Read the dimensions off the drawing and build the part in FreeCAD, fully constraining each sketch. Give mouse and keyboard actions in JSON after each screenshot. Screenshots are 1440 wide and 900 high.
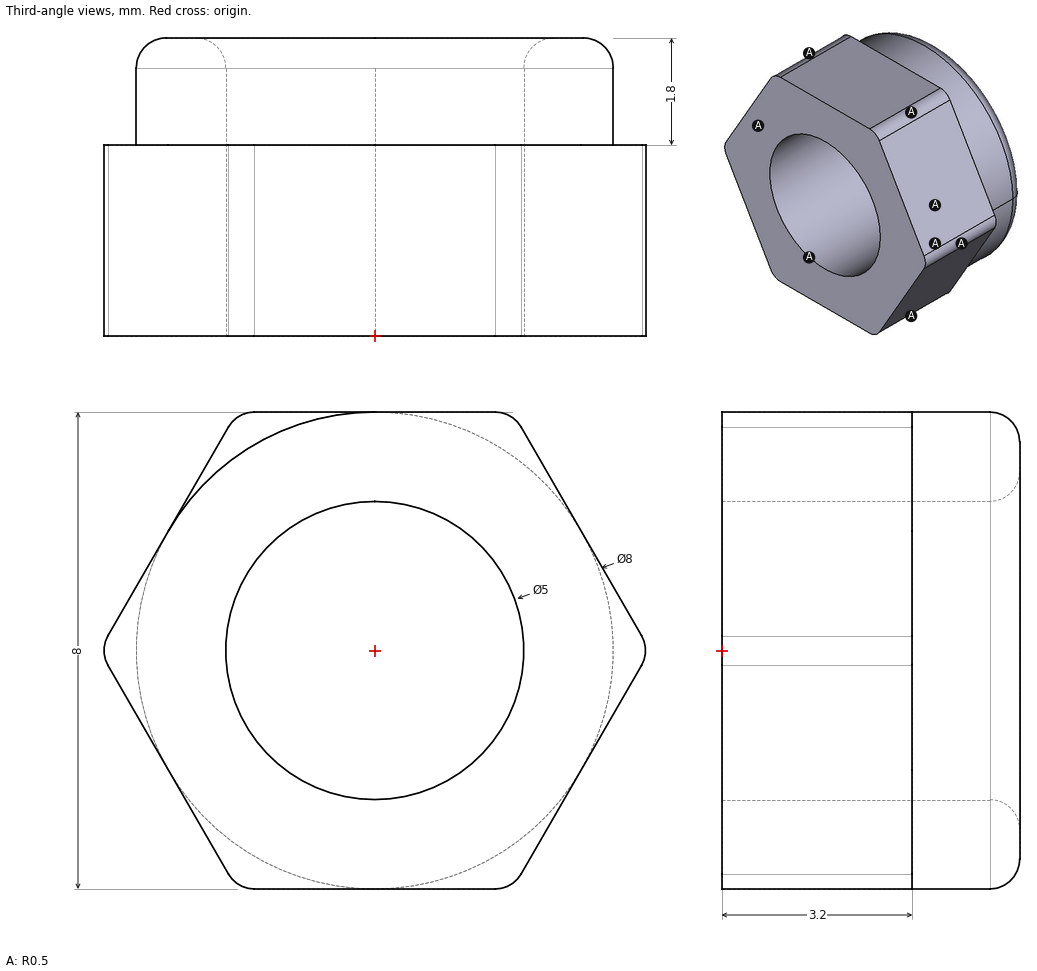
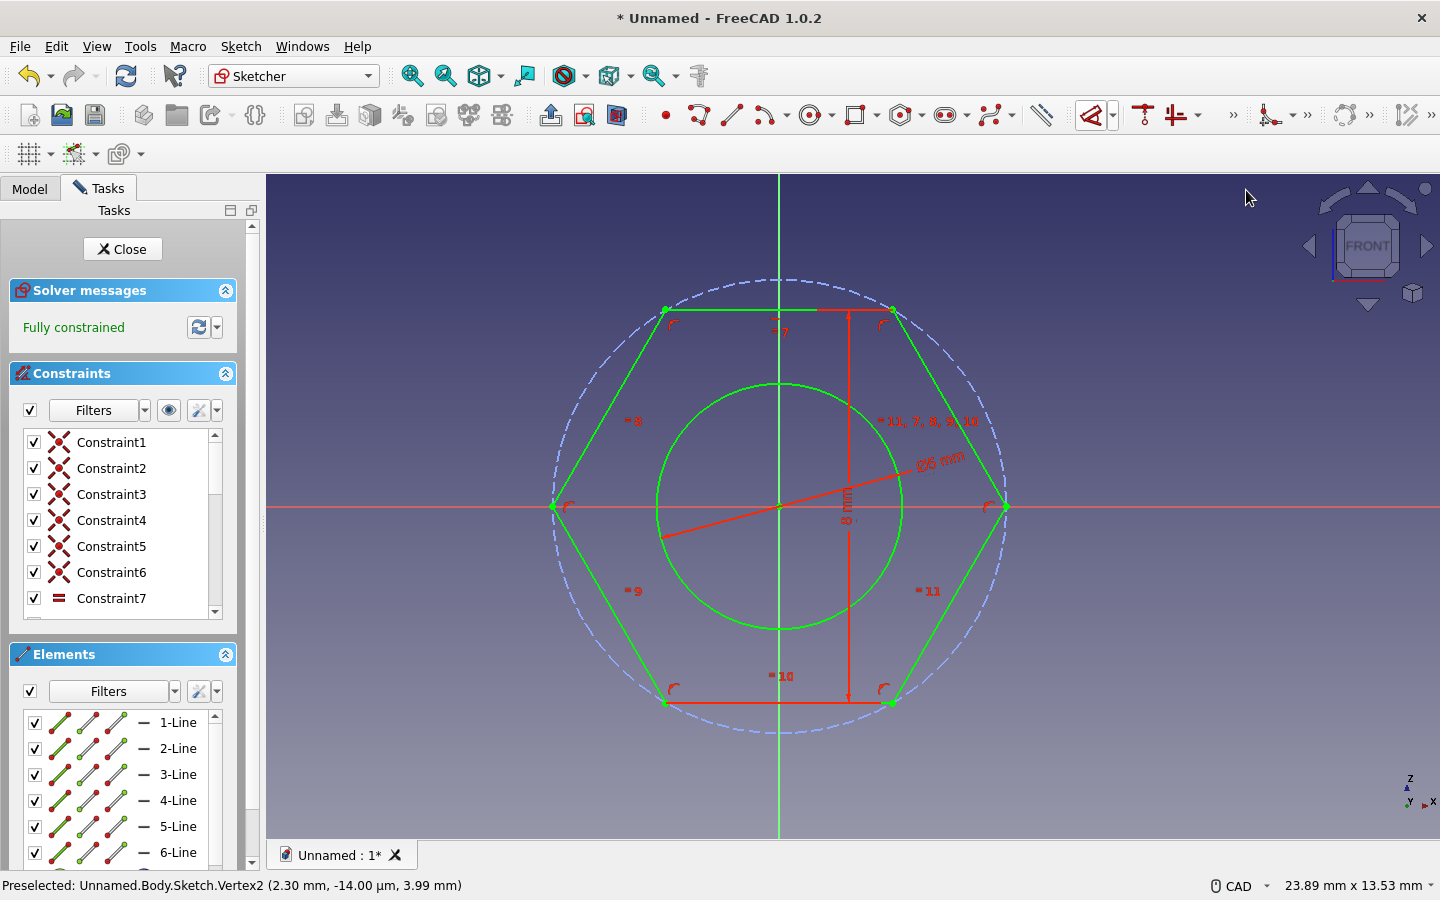
{"action": "left_click", "coordinate": [123, 249]}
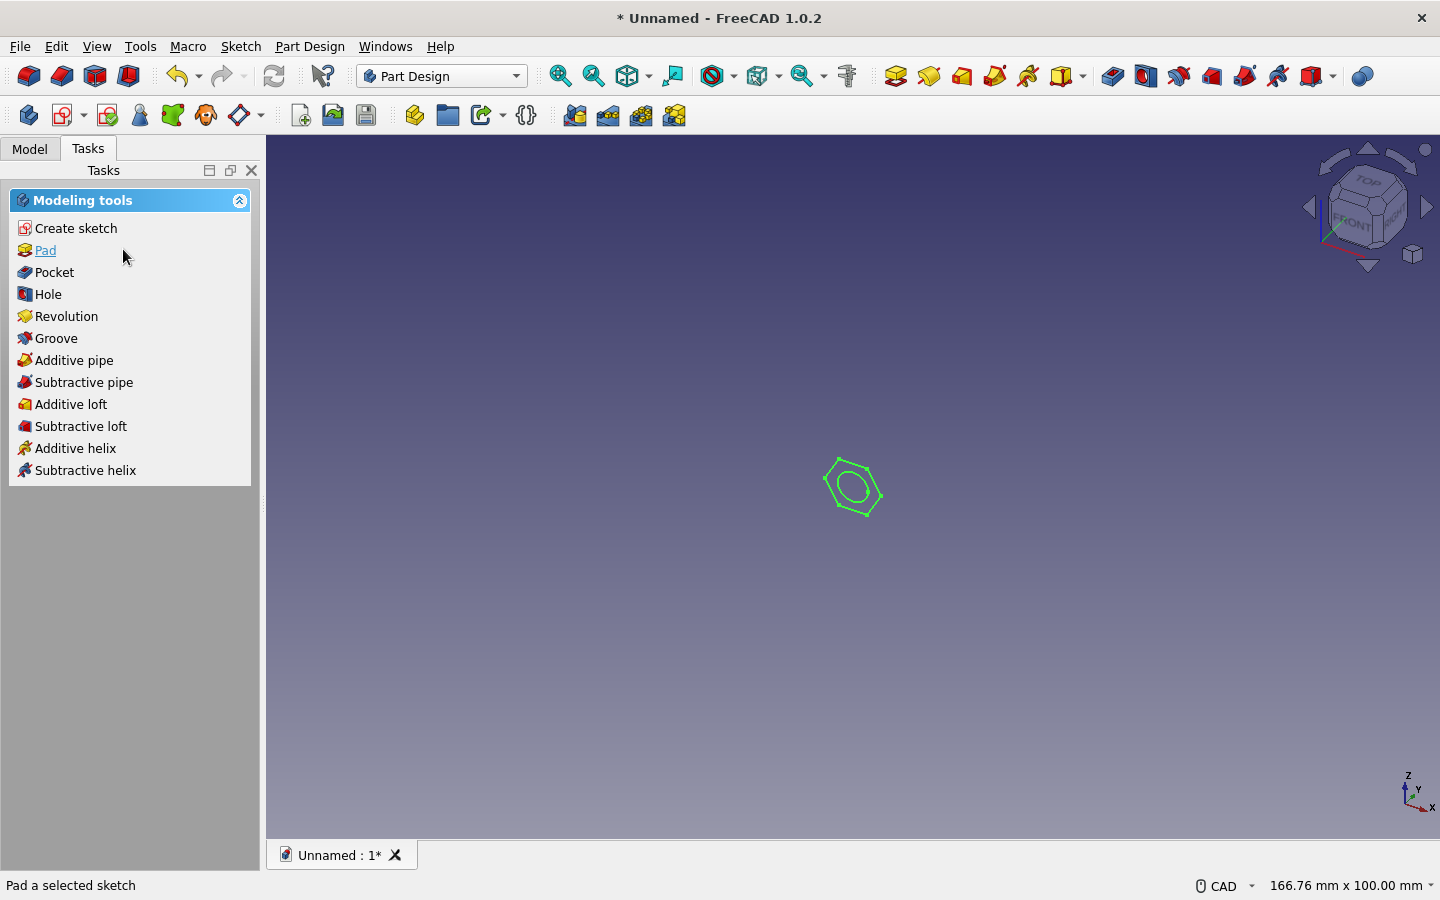
{"action": "left_click", "coordinate": [896, 76]}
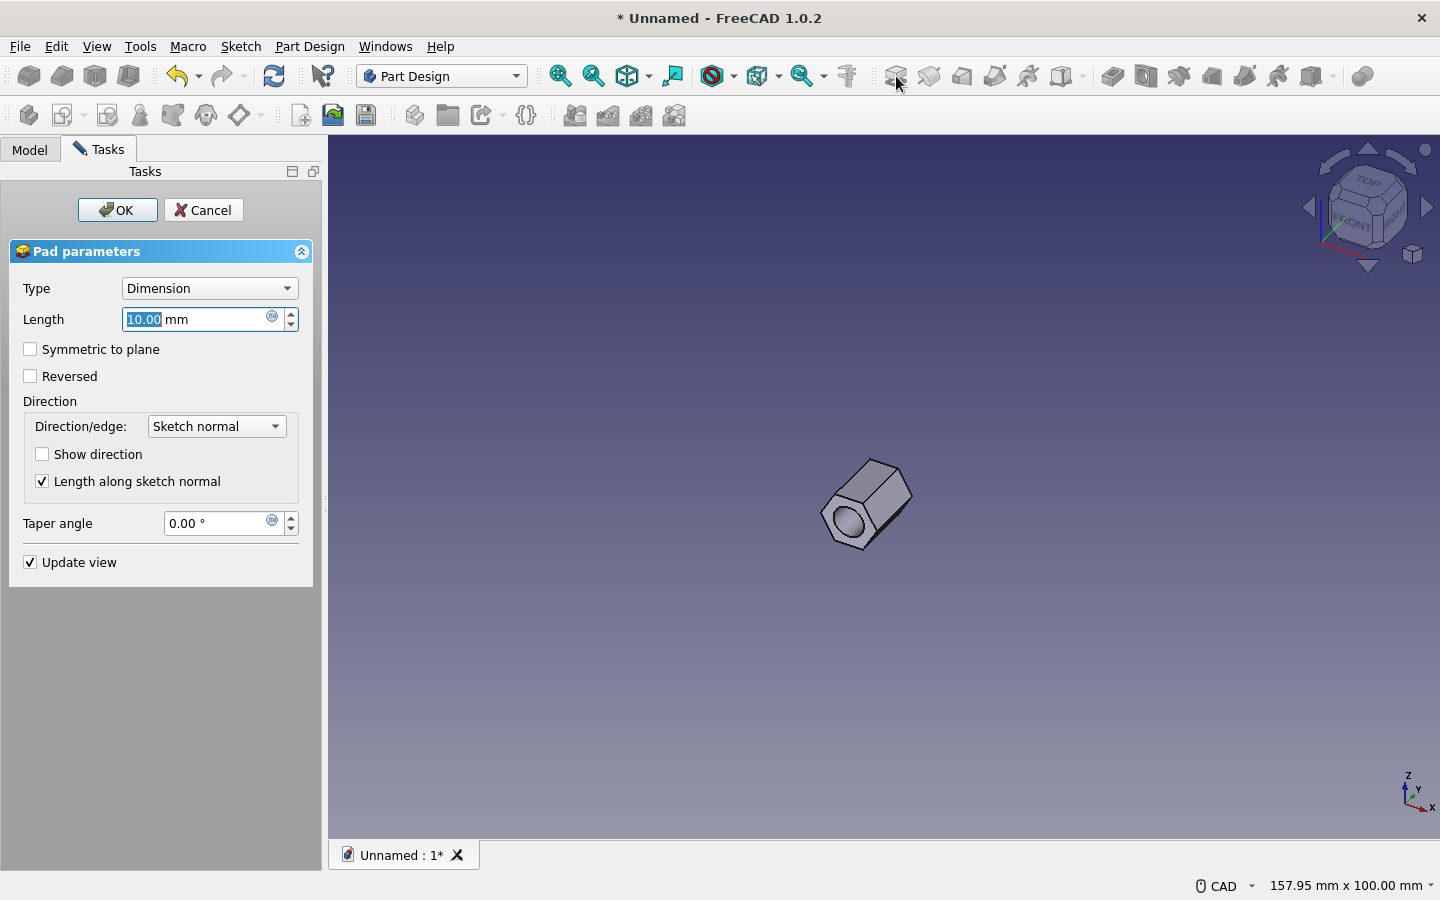
{"action": "type", "text": "3.2"}
{"action": "key", "text": "Tab"}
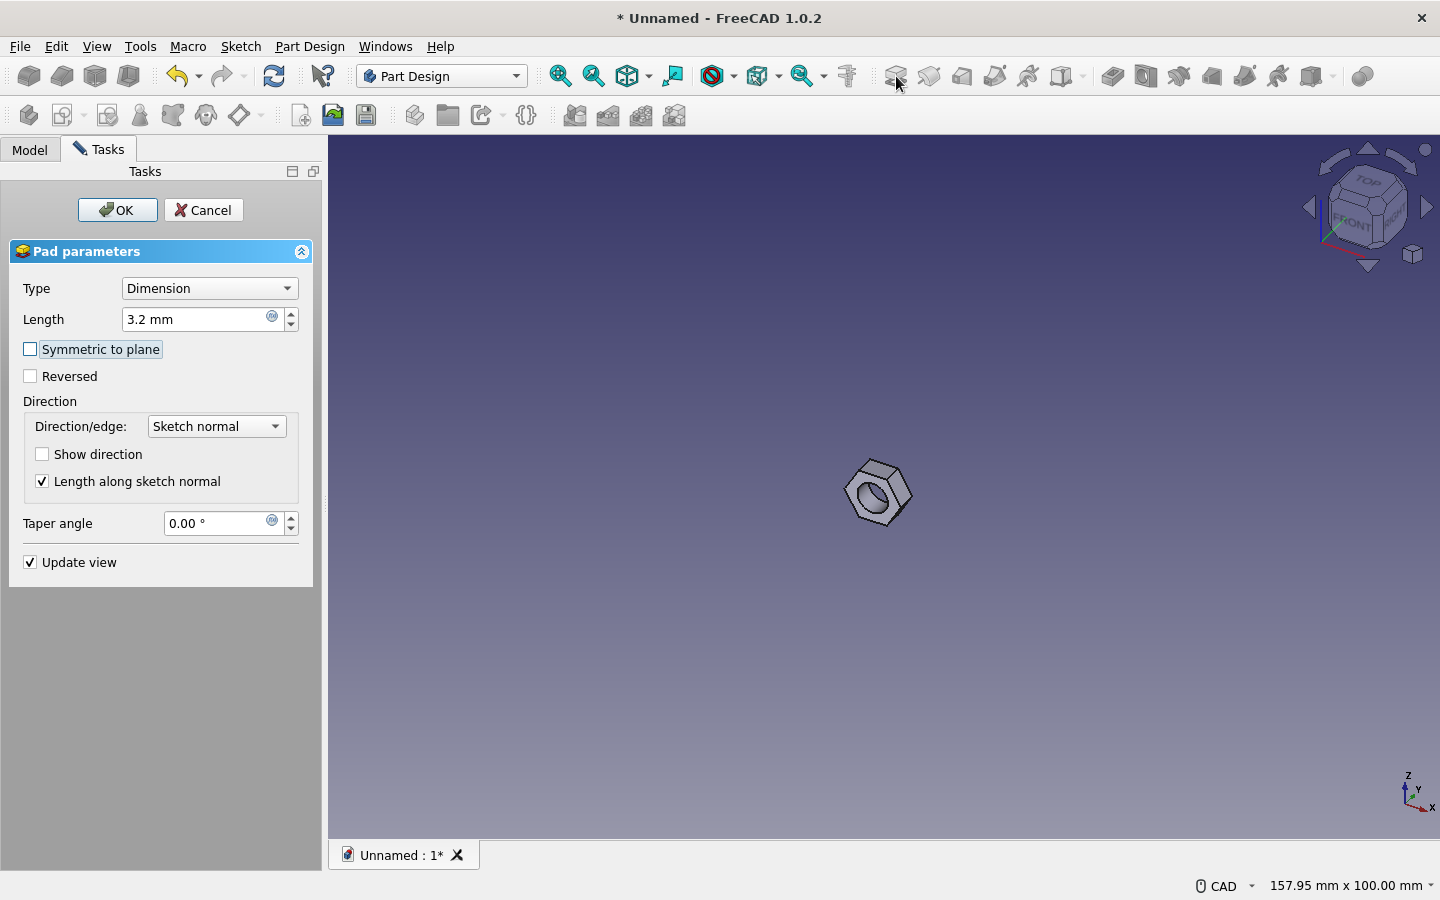
{"action": "left_click", "coordinate": [31, 376]}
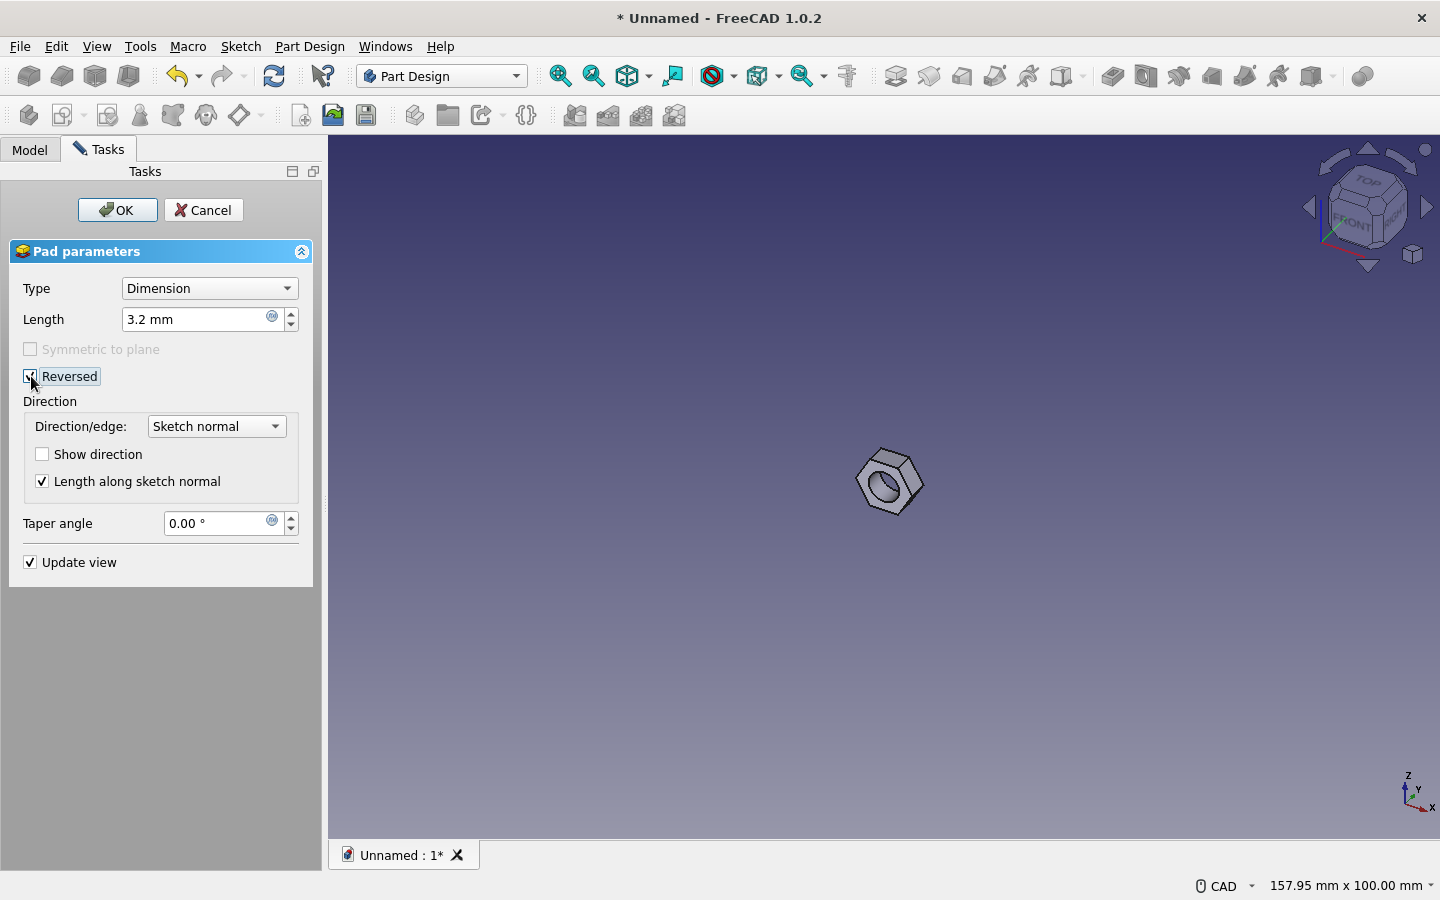
{"action": "left_click", "coordinate": [118, 210]}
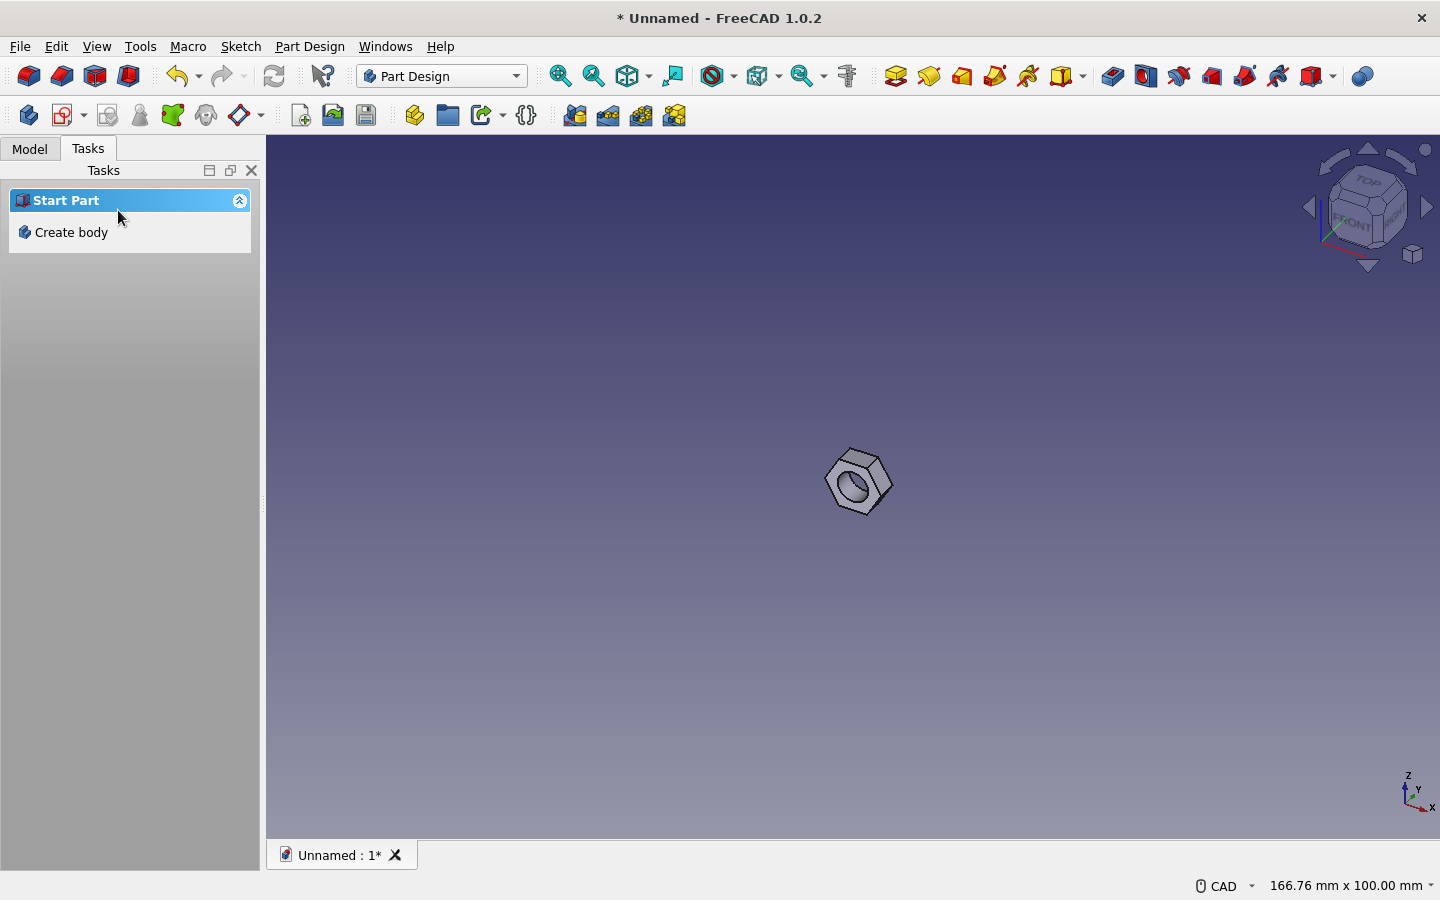
{"action": "key", "text": "v f"}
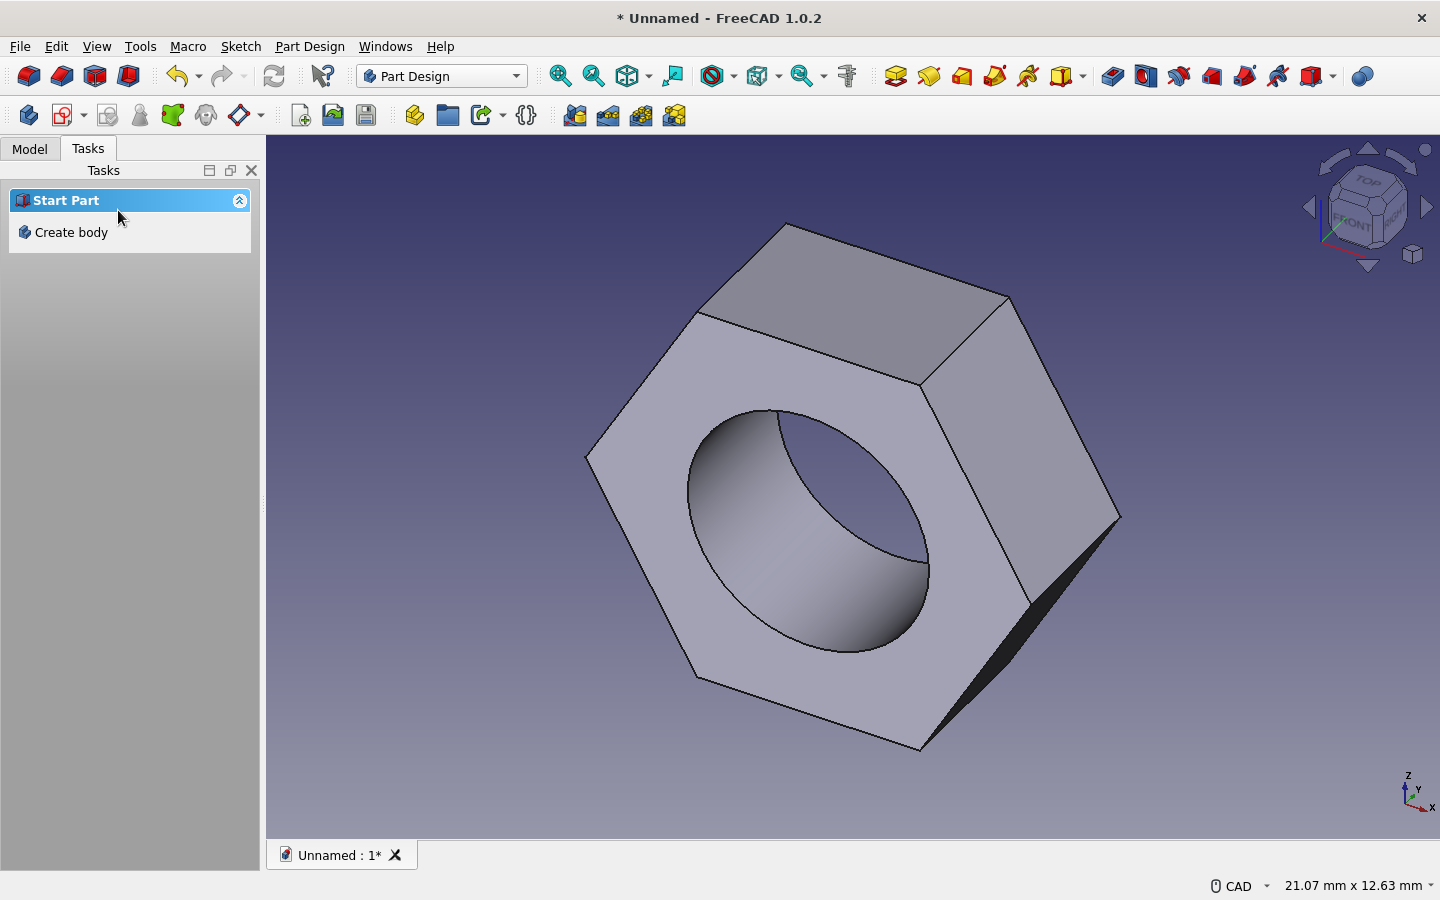
{"action": "key", "text": "4"}